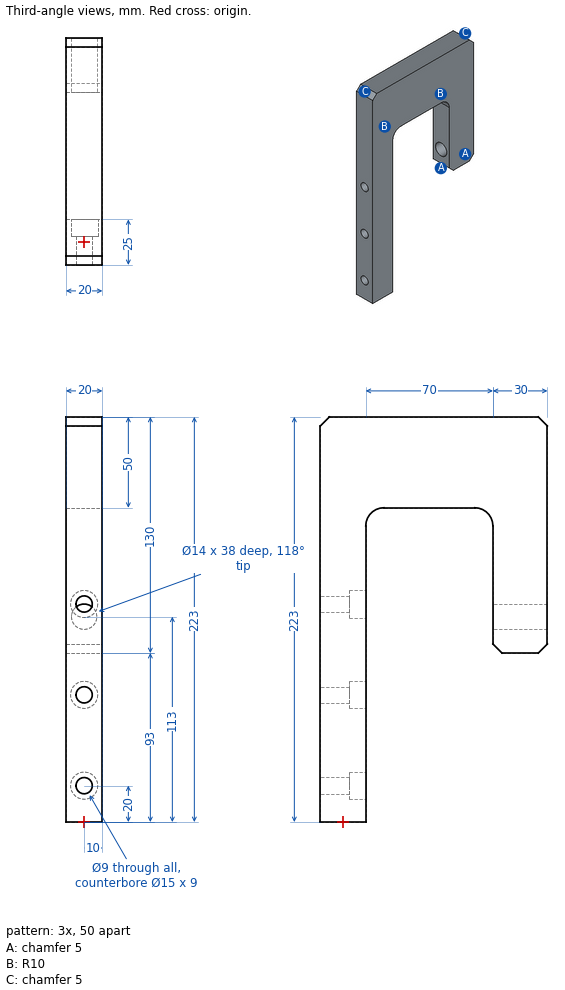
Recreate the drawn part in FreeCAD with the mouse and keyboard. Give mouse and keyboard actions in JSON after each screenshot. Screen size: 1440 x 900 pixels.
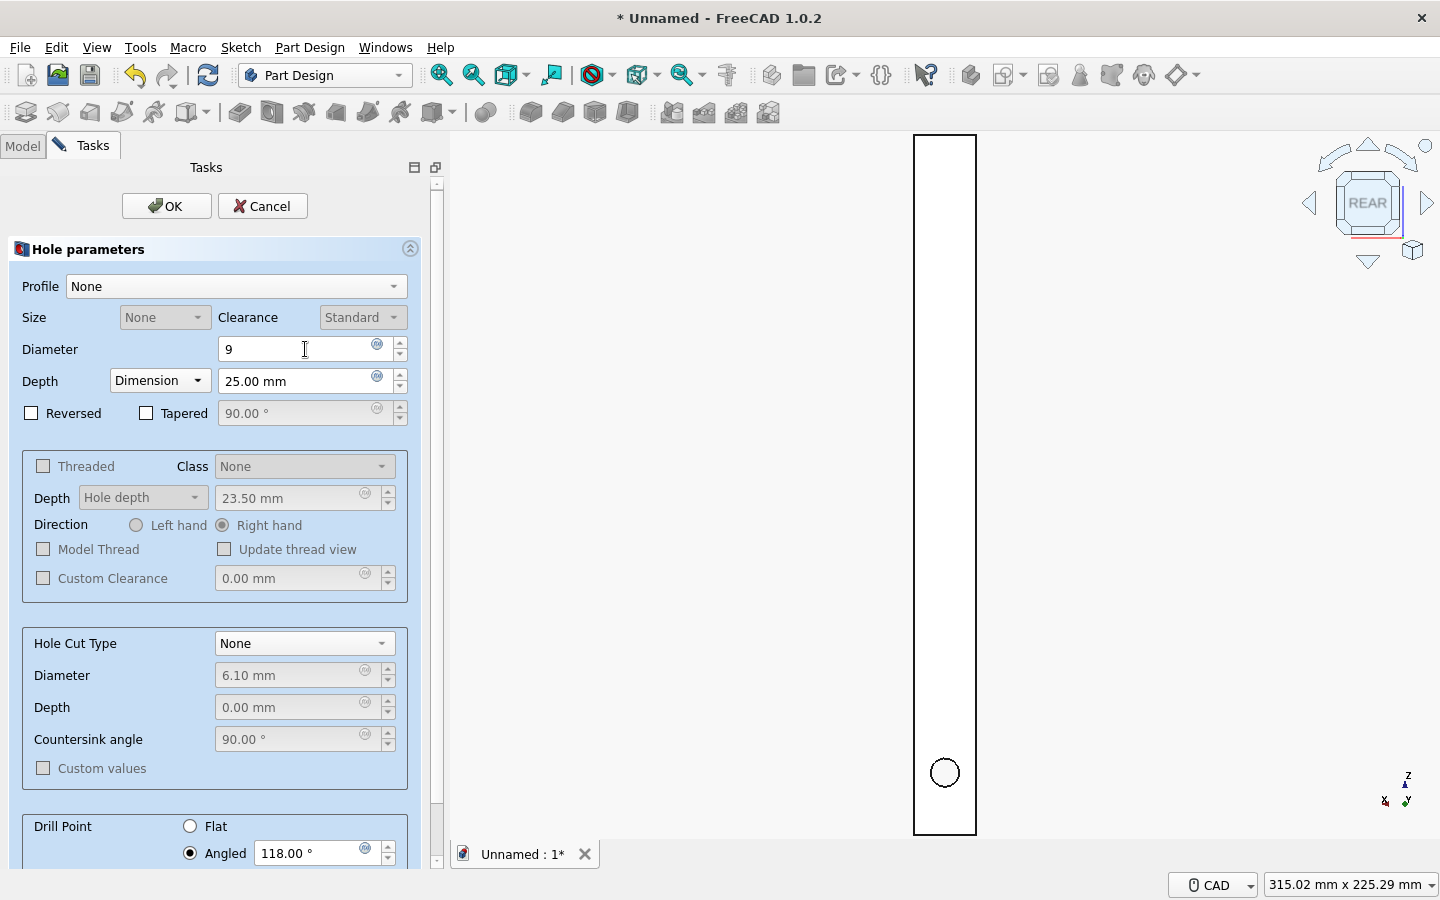
{"action": "left_click", "coordinate": [161, 380]}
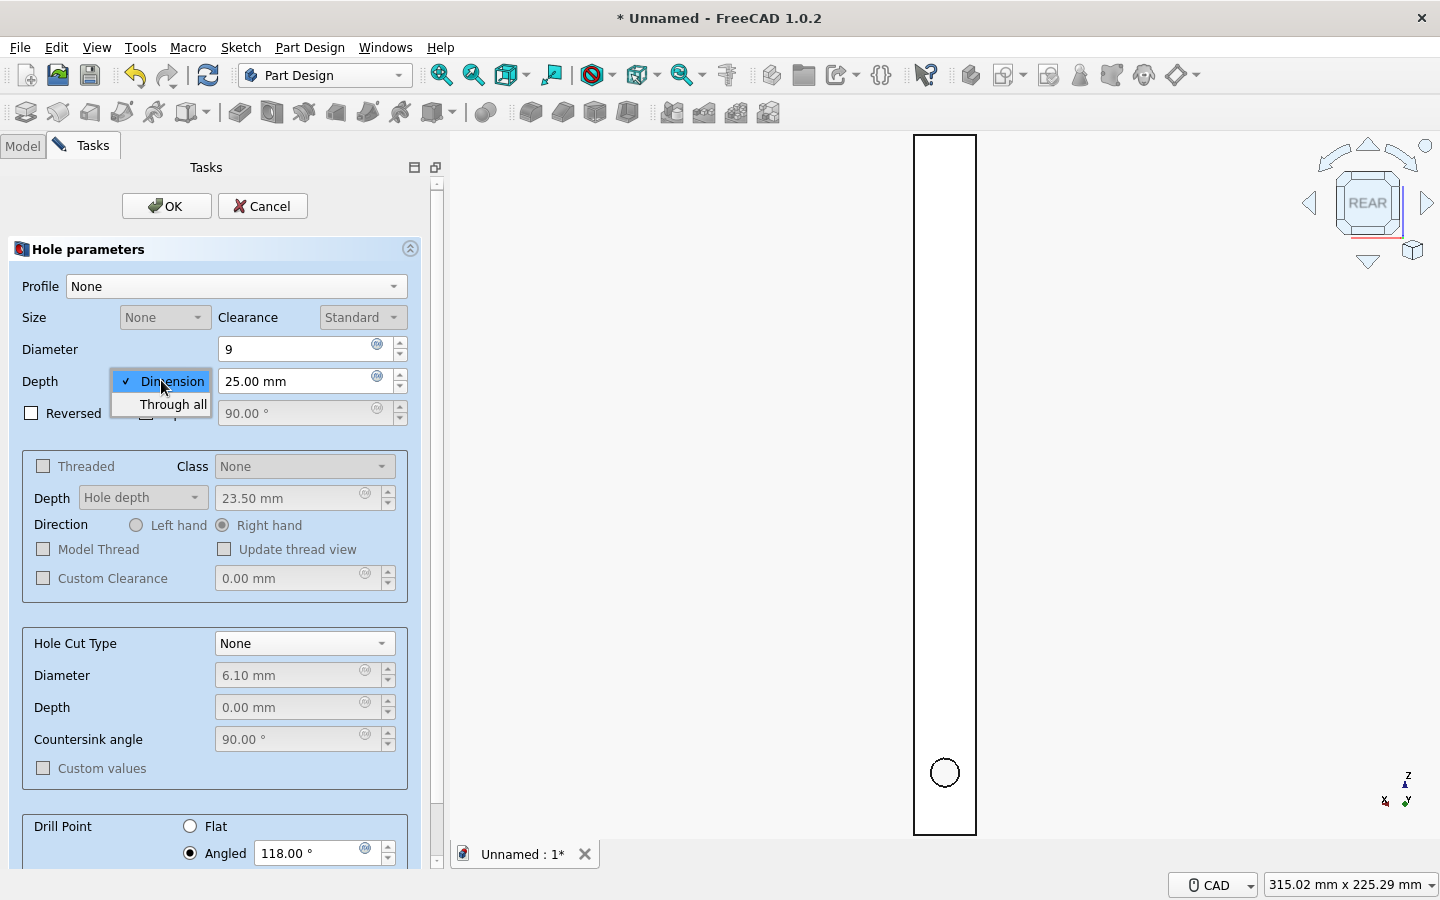
{"action": "left_click", "coordinate": [160, 404]}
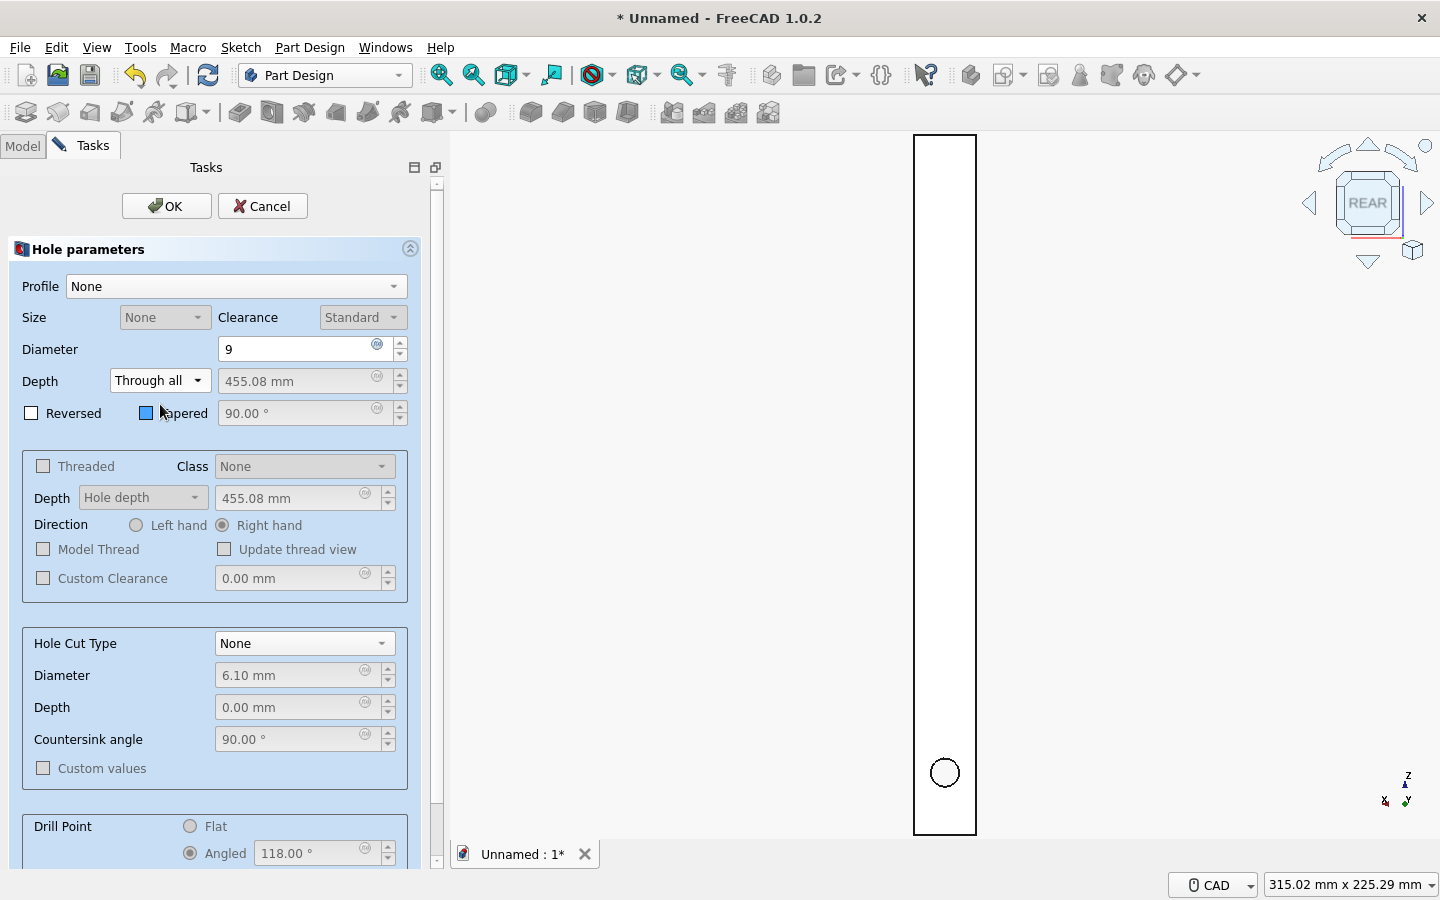
{"action": "left_click", "coordinate": [306, 644]}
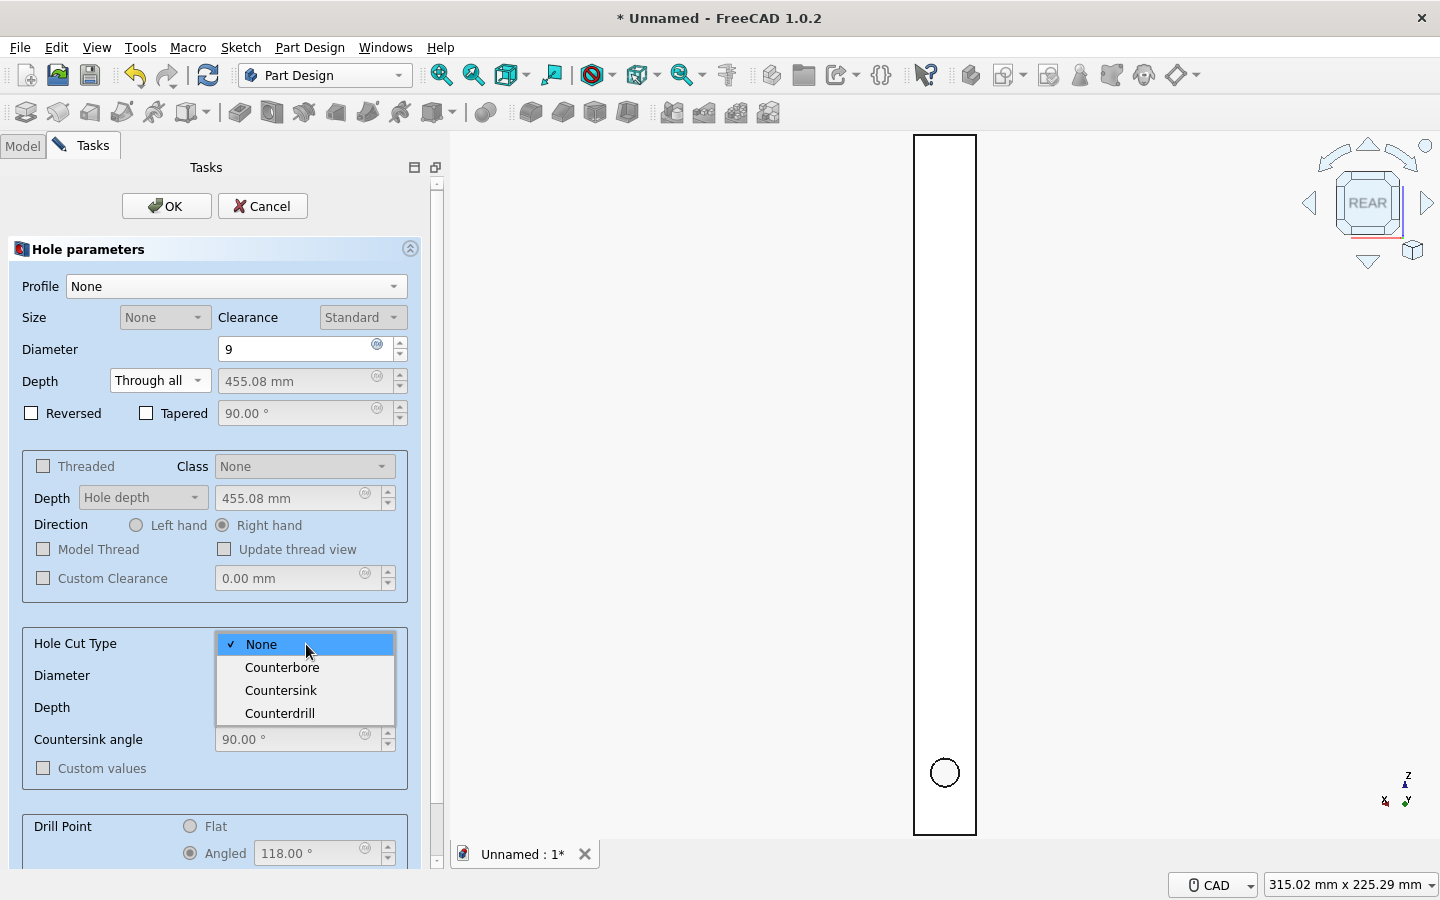
{"action": "left_click", "coordinate": [304, 668]}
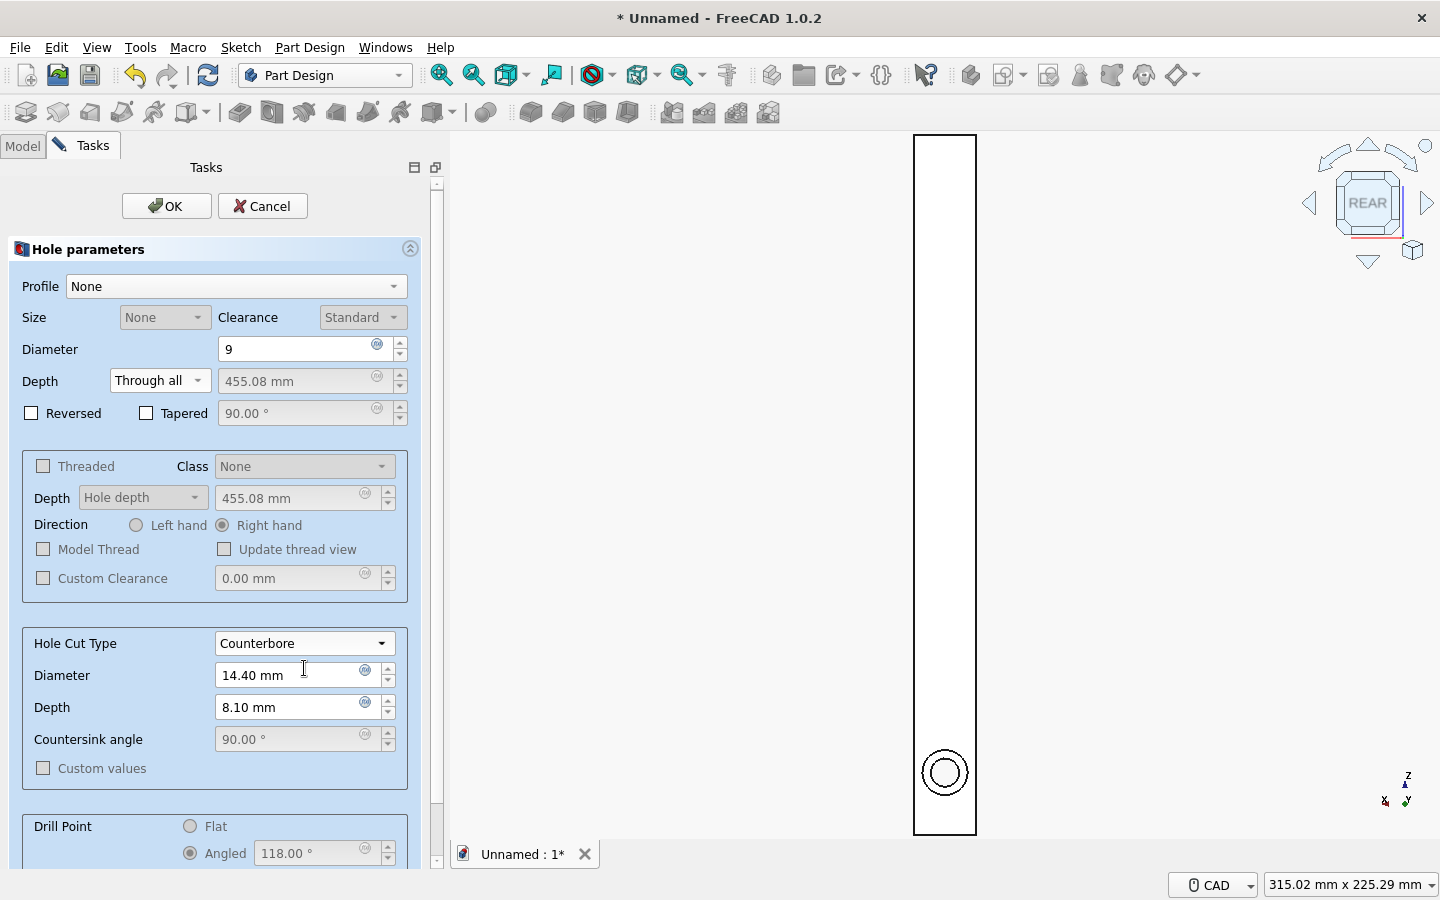
{"action": "triple_click", "coordinate": [298, 675]}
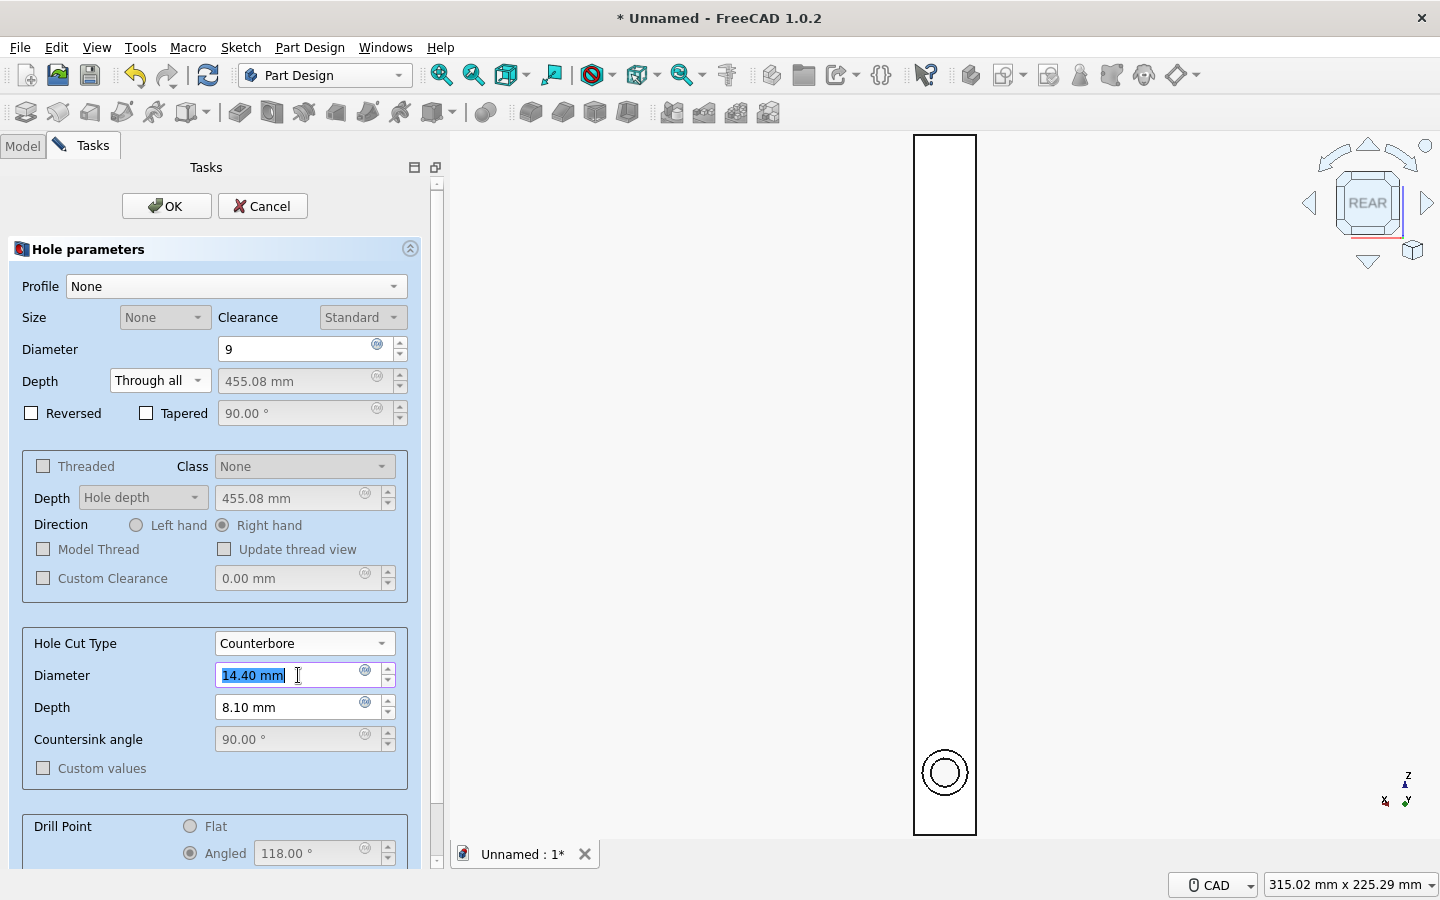
{"action": "type", "text": "15"}
{"action": "key", "text": "Tab"}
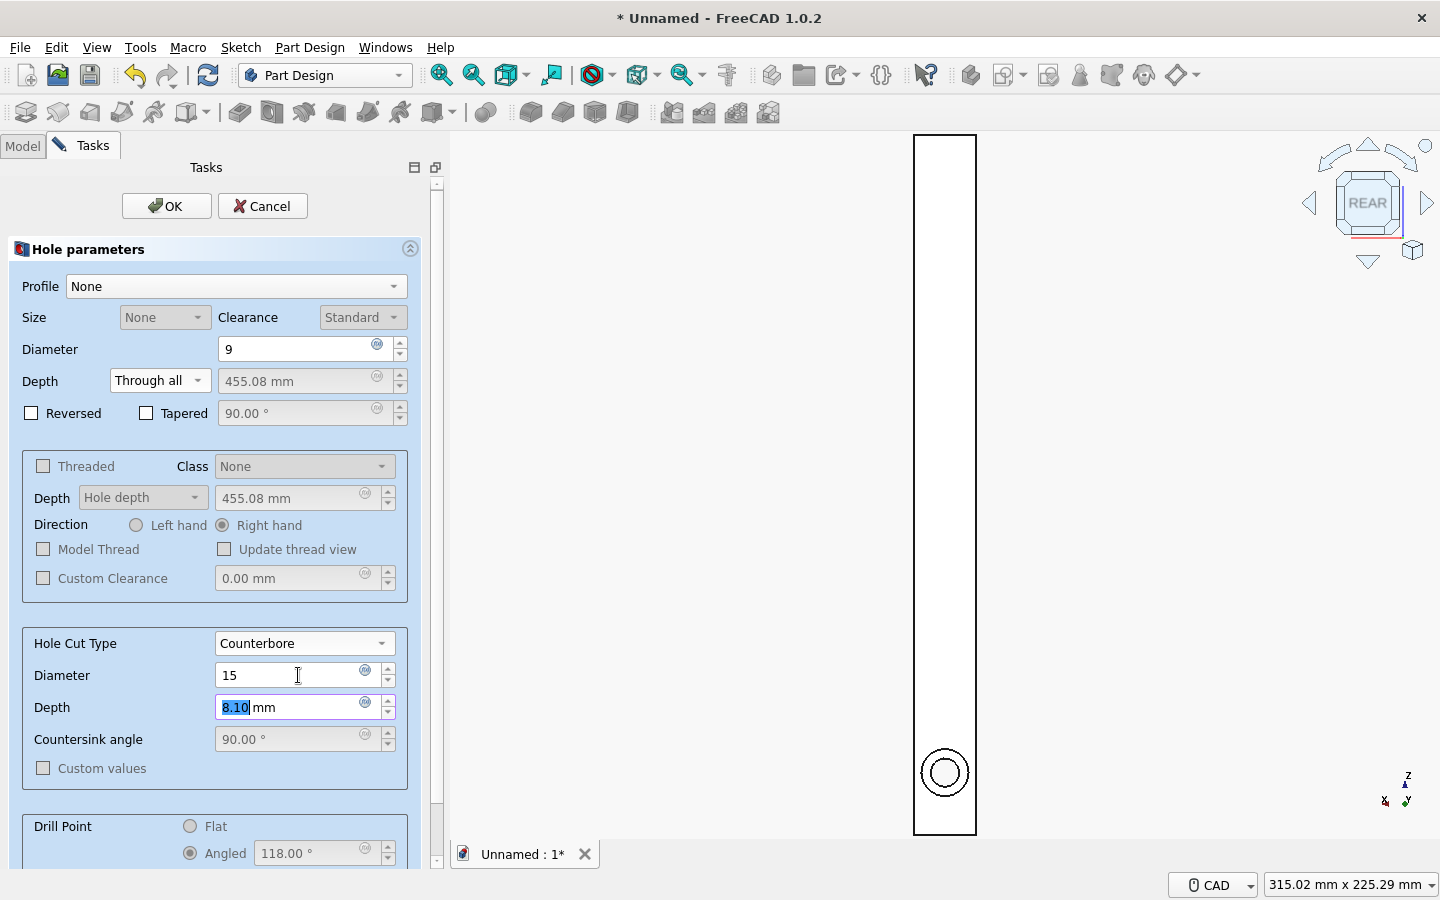
{"action": "type", "text": "9"}
{"action": "key", "text": "Tab"}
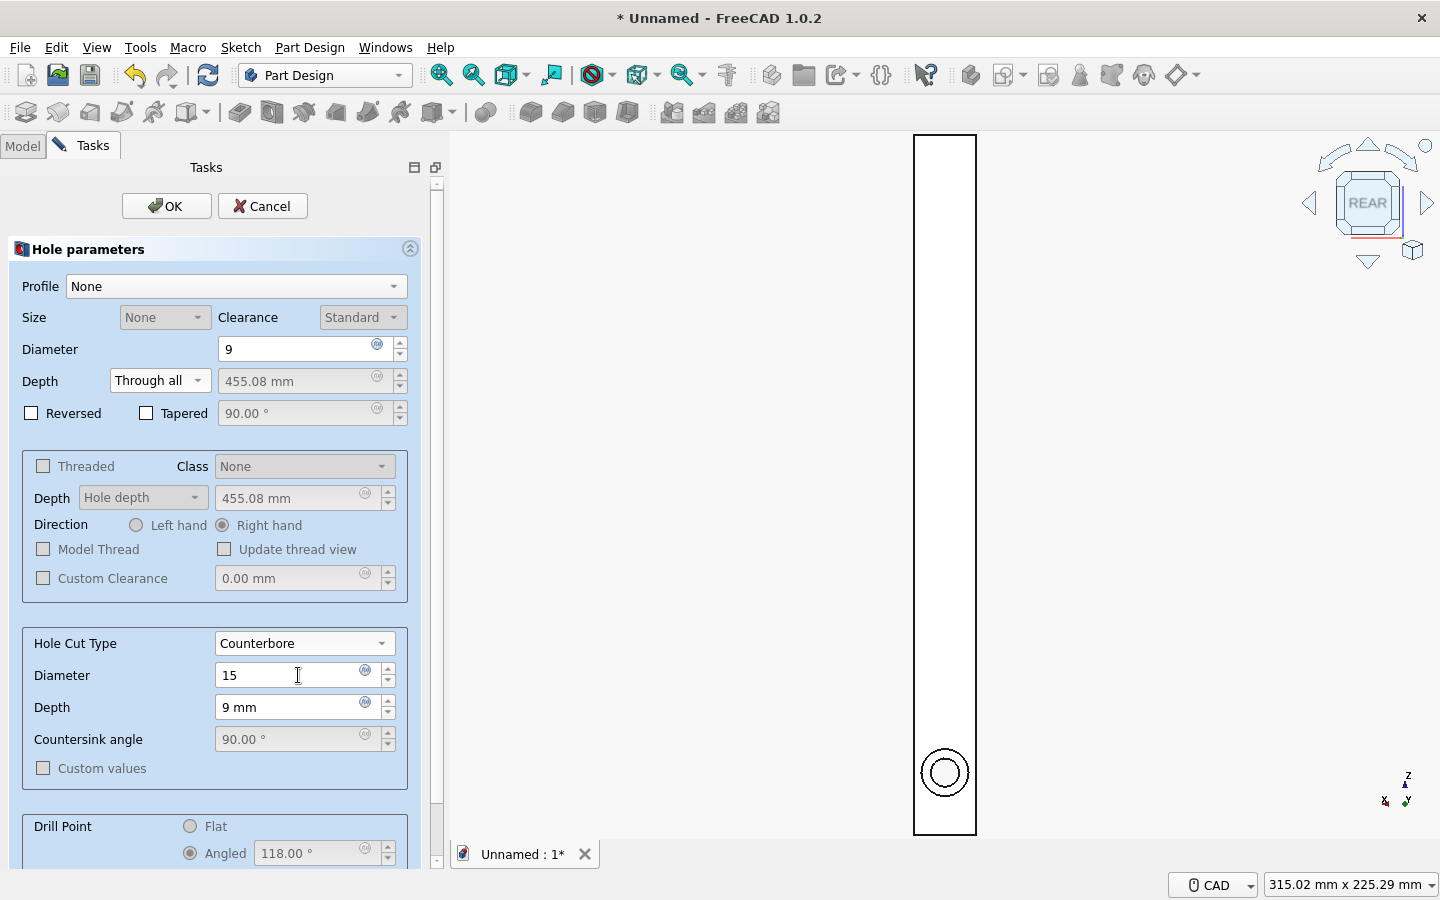
{"action": "left_click", "coordinate": [167, 206]}